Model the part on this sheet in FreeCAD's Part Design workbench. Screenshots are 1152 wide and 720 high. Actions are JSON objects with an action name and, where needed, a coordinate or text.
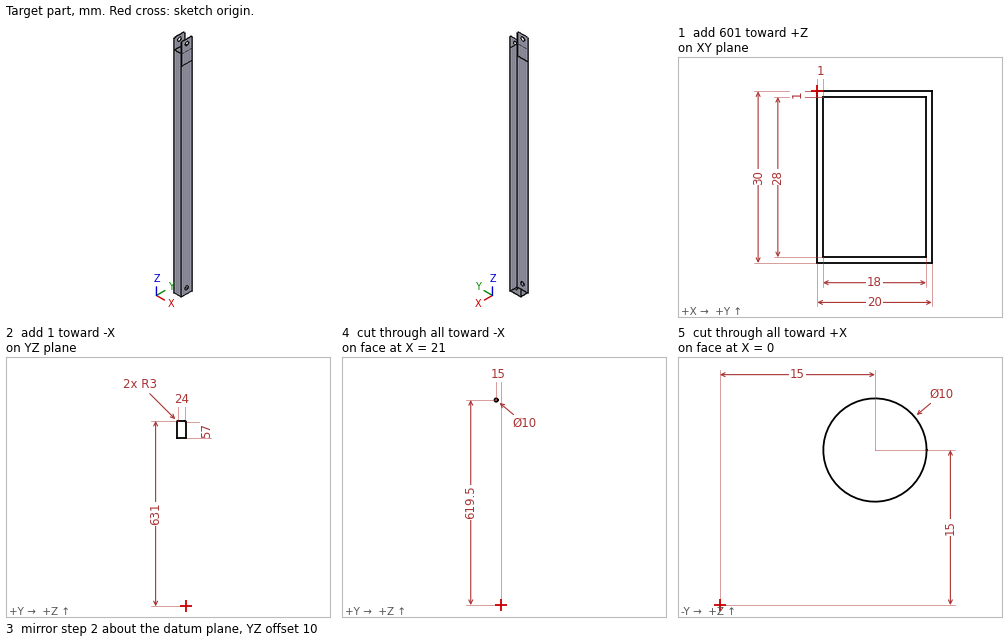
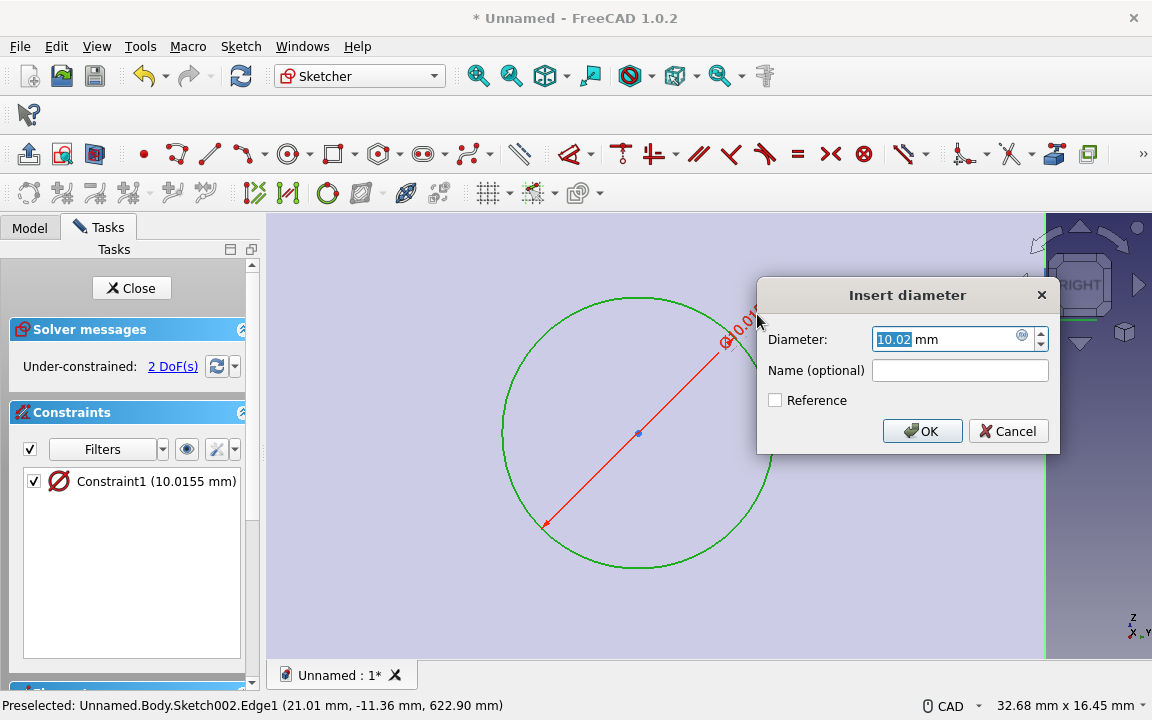
{"action": "type", "text": "10"}
{"action": "key", "text": "Return"}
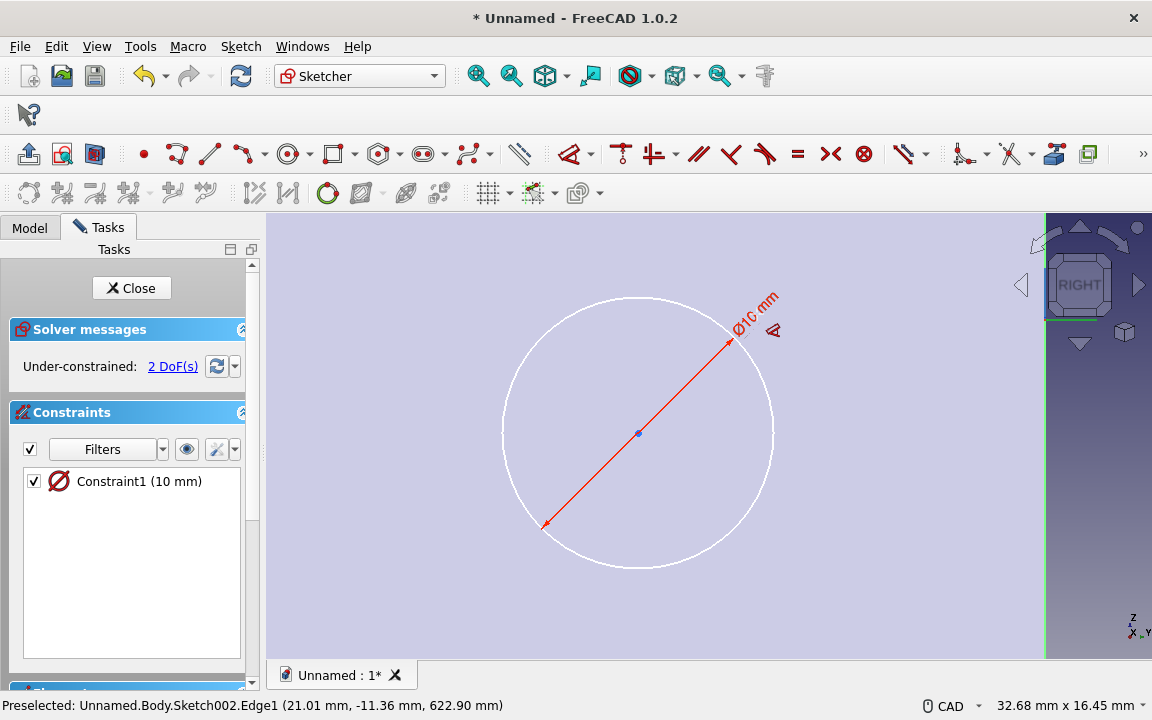
{"action": "left_click", "coordinate": [638, 433]}
{"action": "left_click", "coordinate": [813, 399]}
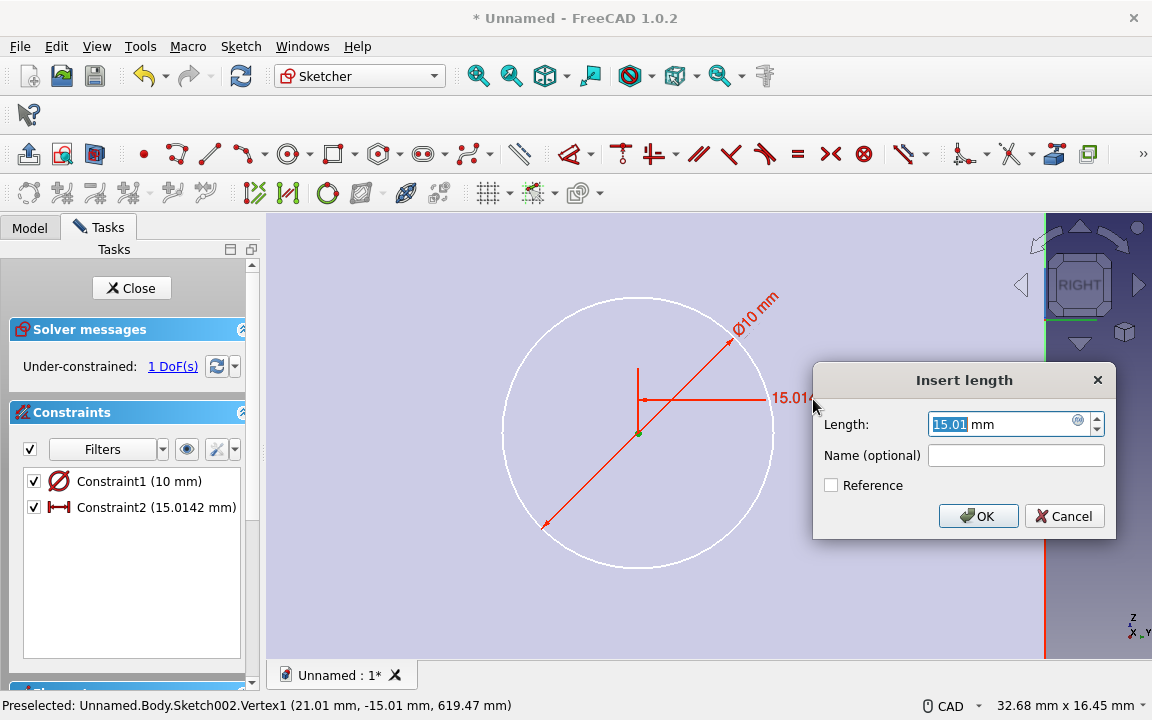
{"action": "type", "text": "15"}
{"action": "key", "text": "Return"}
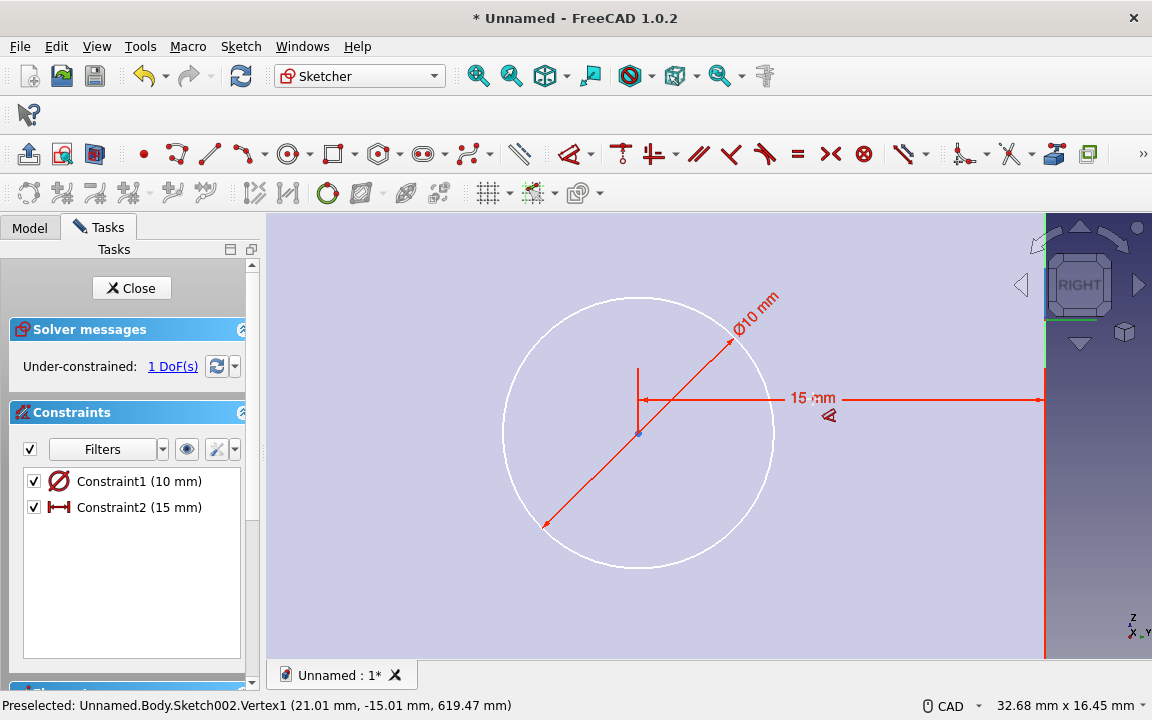
{"action": "left_click", "coordinate": [638, 433]}
{"action": "left_click", "coordinate": [604, 532]}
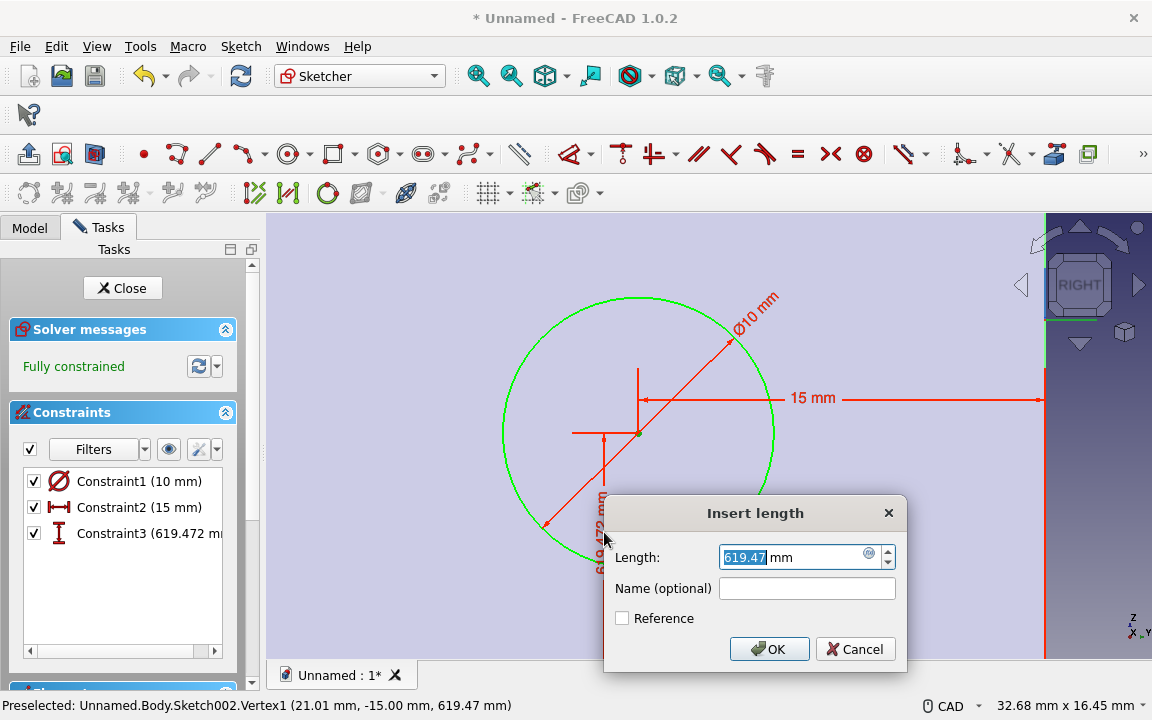
{"action": "type", "text": "619.5"}
{"action": "key", "text": "Return"}
{"action": "key", "text": "Escape"}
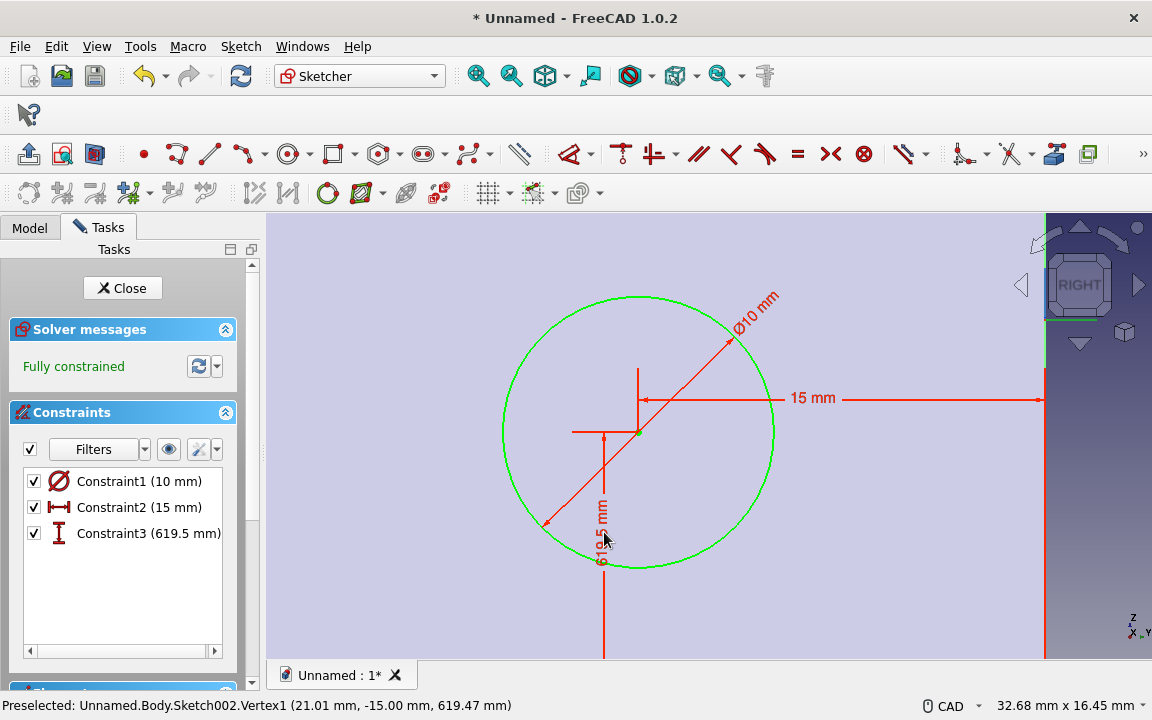
{"action": "left_click", "coordinate": [123, 288]}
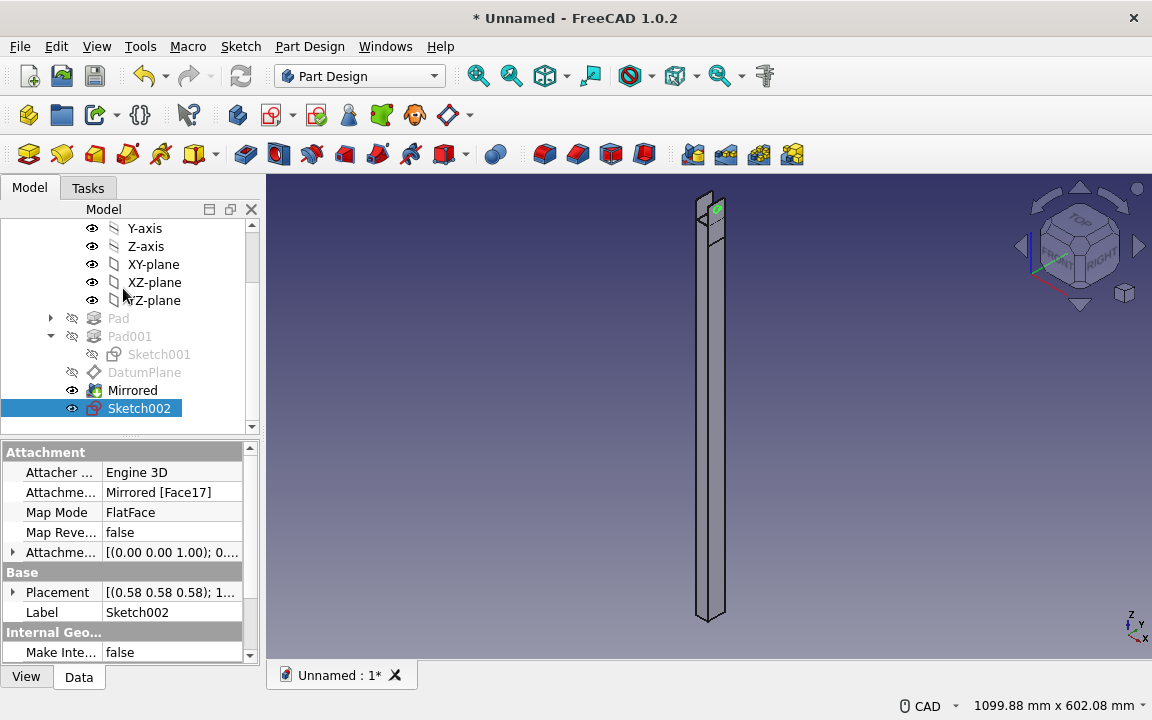
{"action": "left_click", "coordinate": [246, 154]}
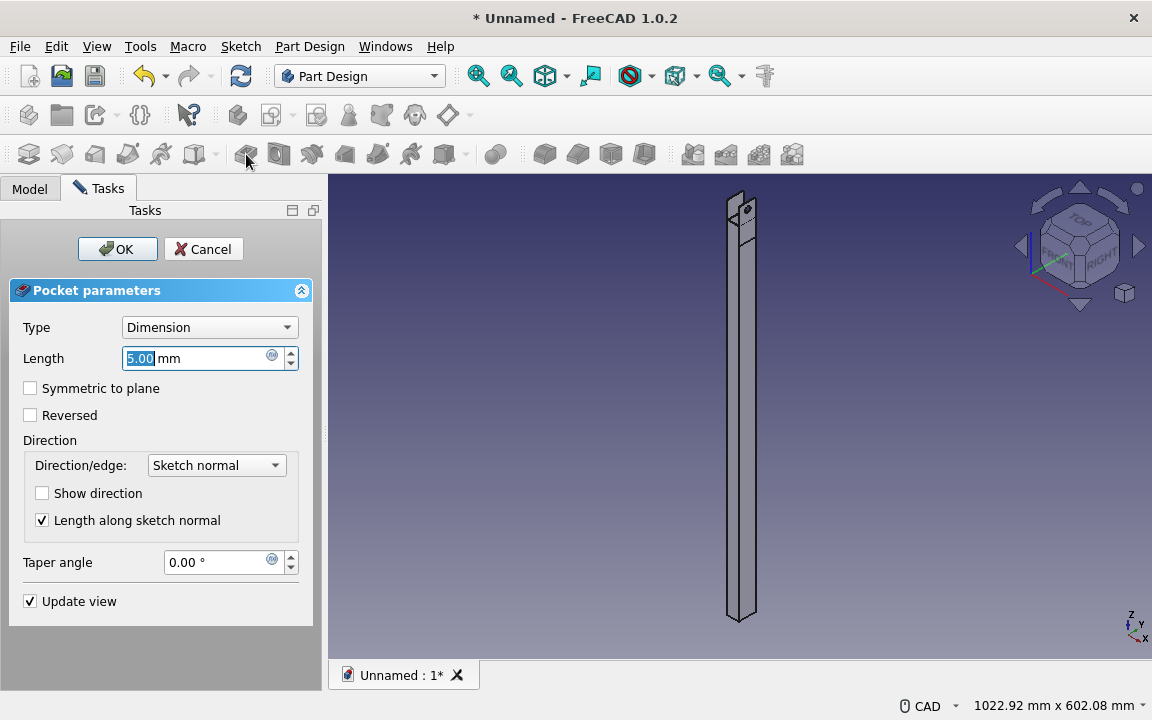
{"action": "left_click", "coordinate": [210, 328]}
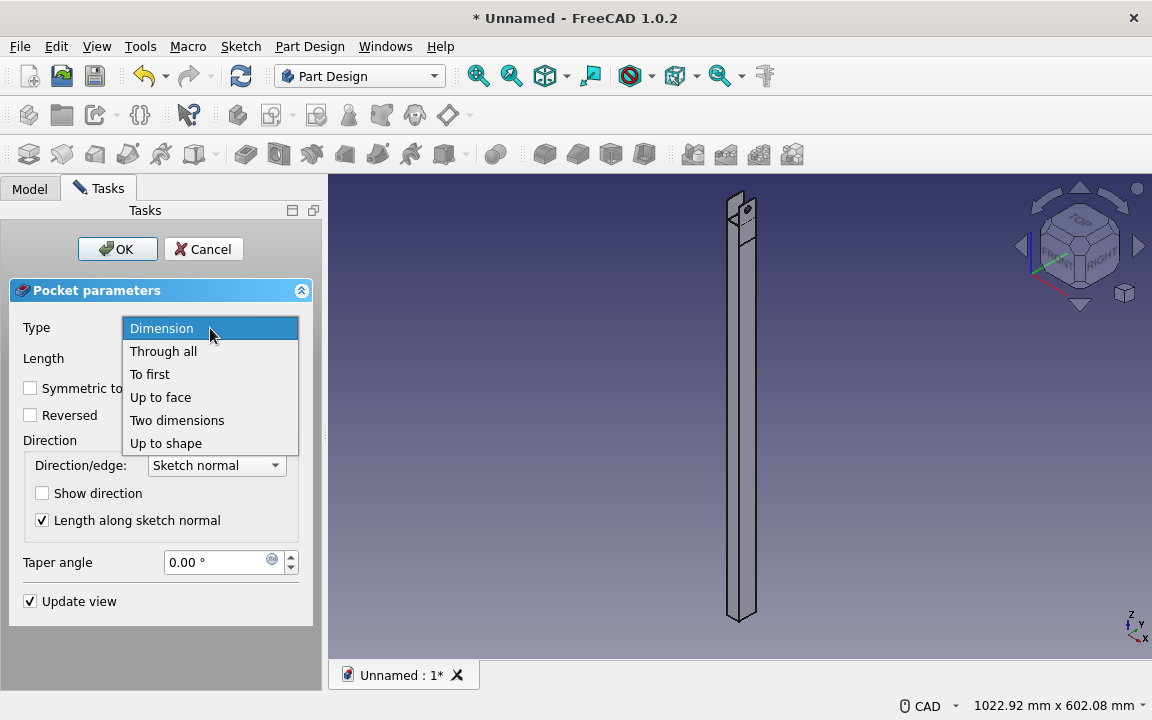
{"action": "left_click", "coordinate": [208, 352]}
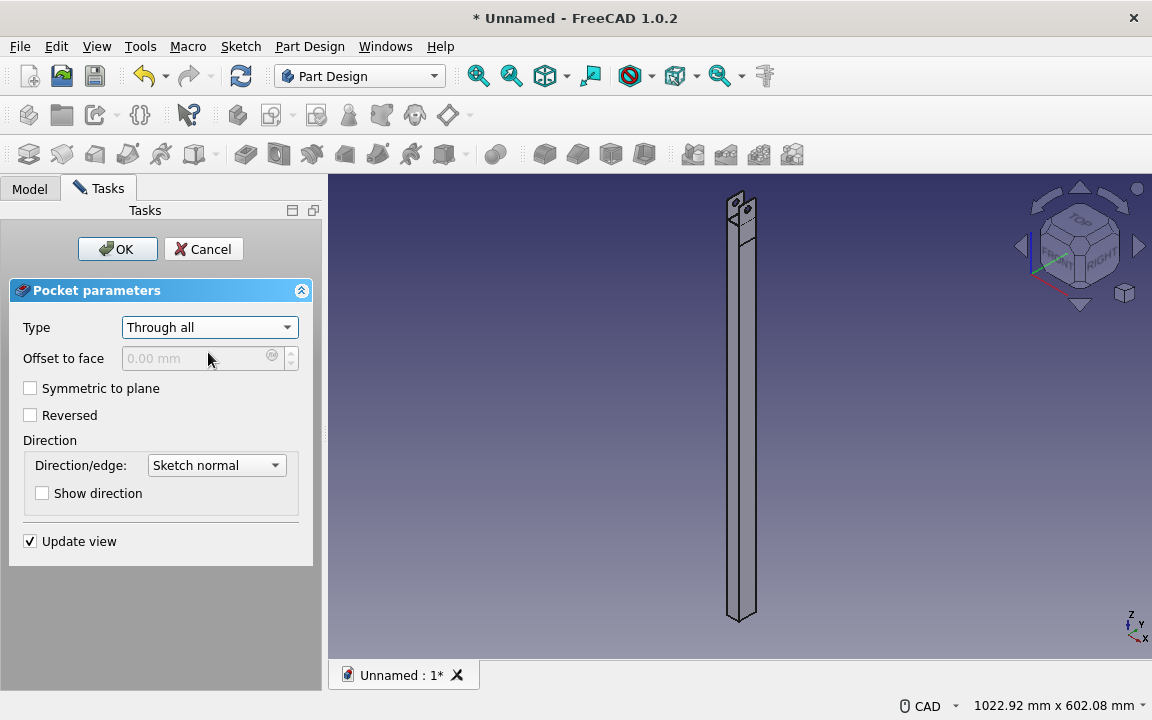
{"action": "left_click", "coordinate": [118, 249]}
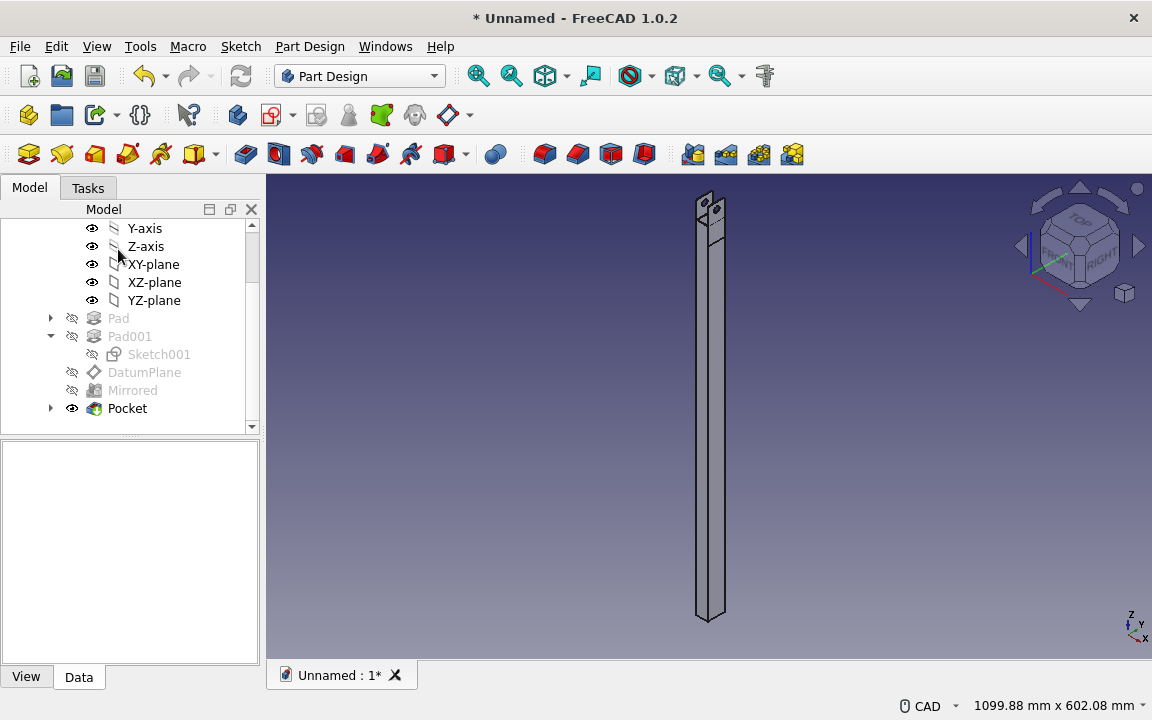
{"action": "key", "text": "6"}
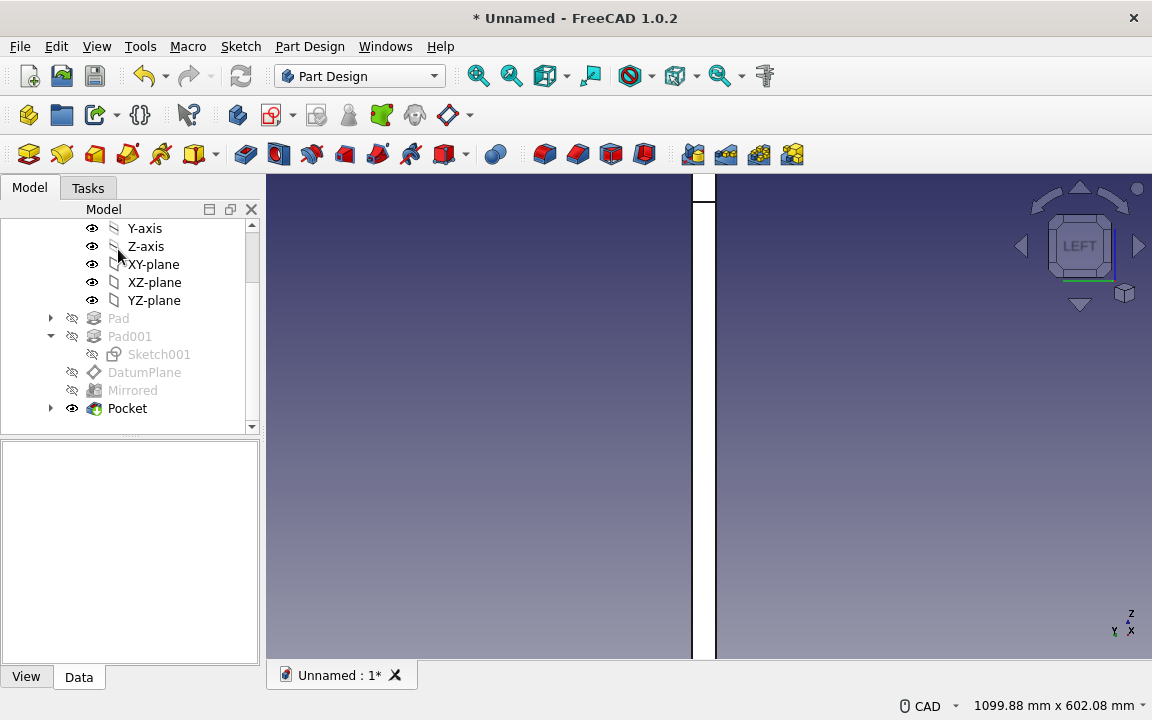
{"action": "key", "text": "v f"}